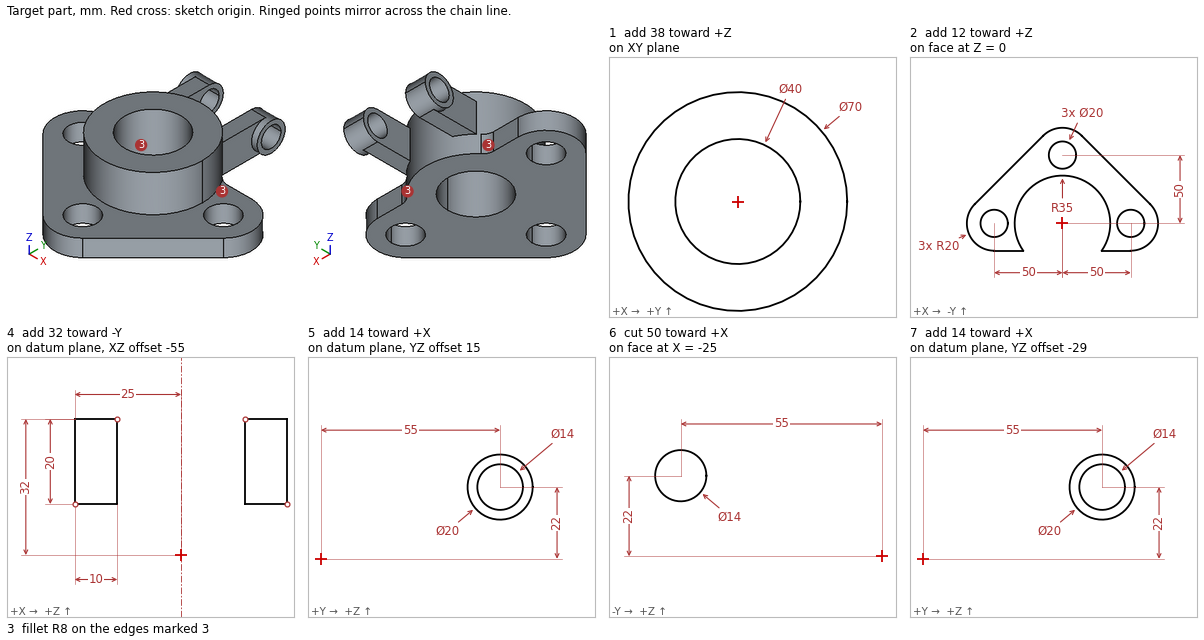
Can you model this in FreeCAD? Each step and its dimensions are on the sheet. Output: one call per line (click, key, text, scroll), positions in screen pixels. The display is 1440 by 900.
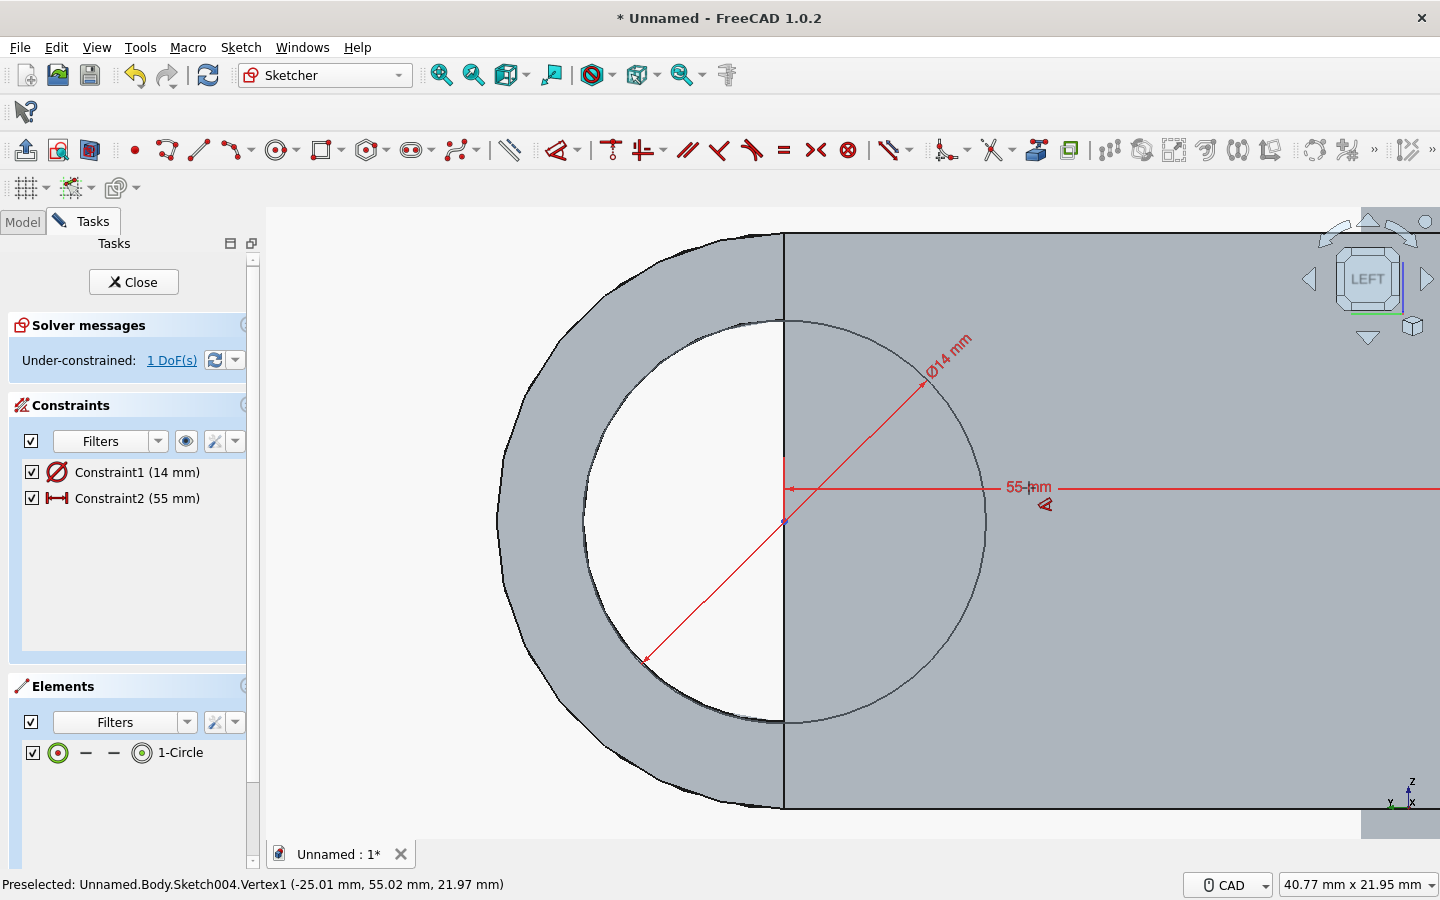
click(784, 522)
click(750, 667)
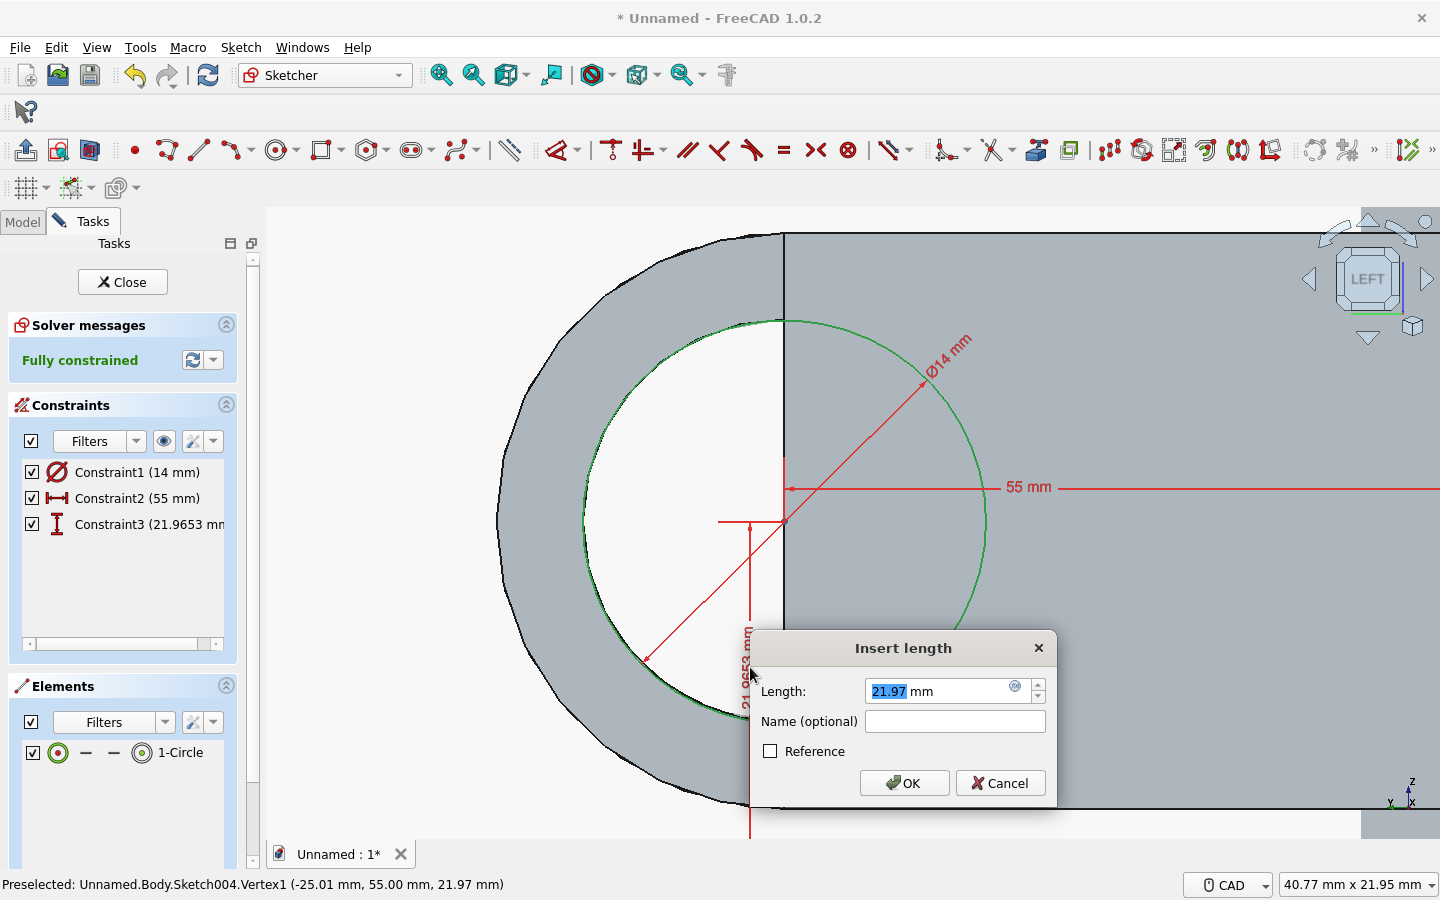
text(22)
key(Return)
key(Escape)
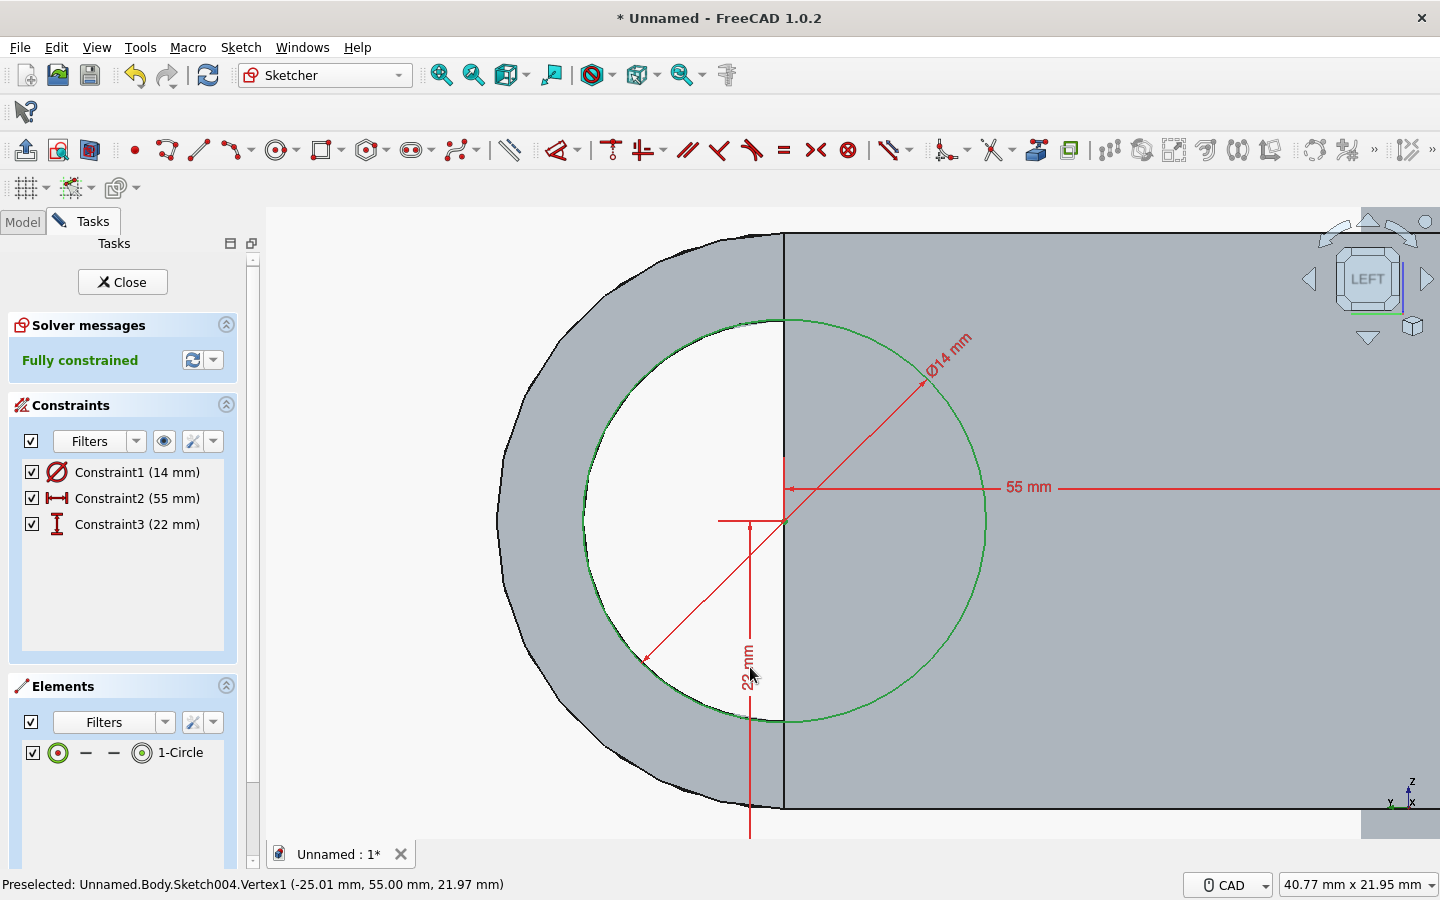
click(123, 282)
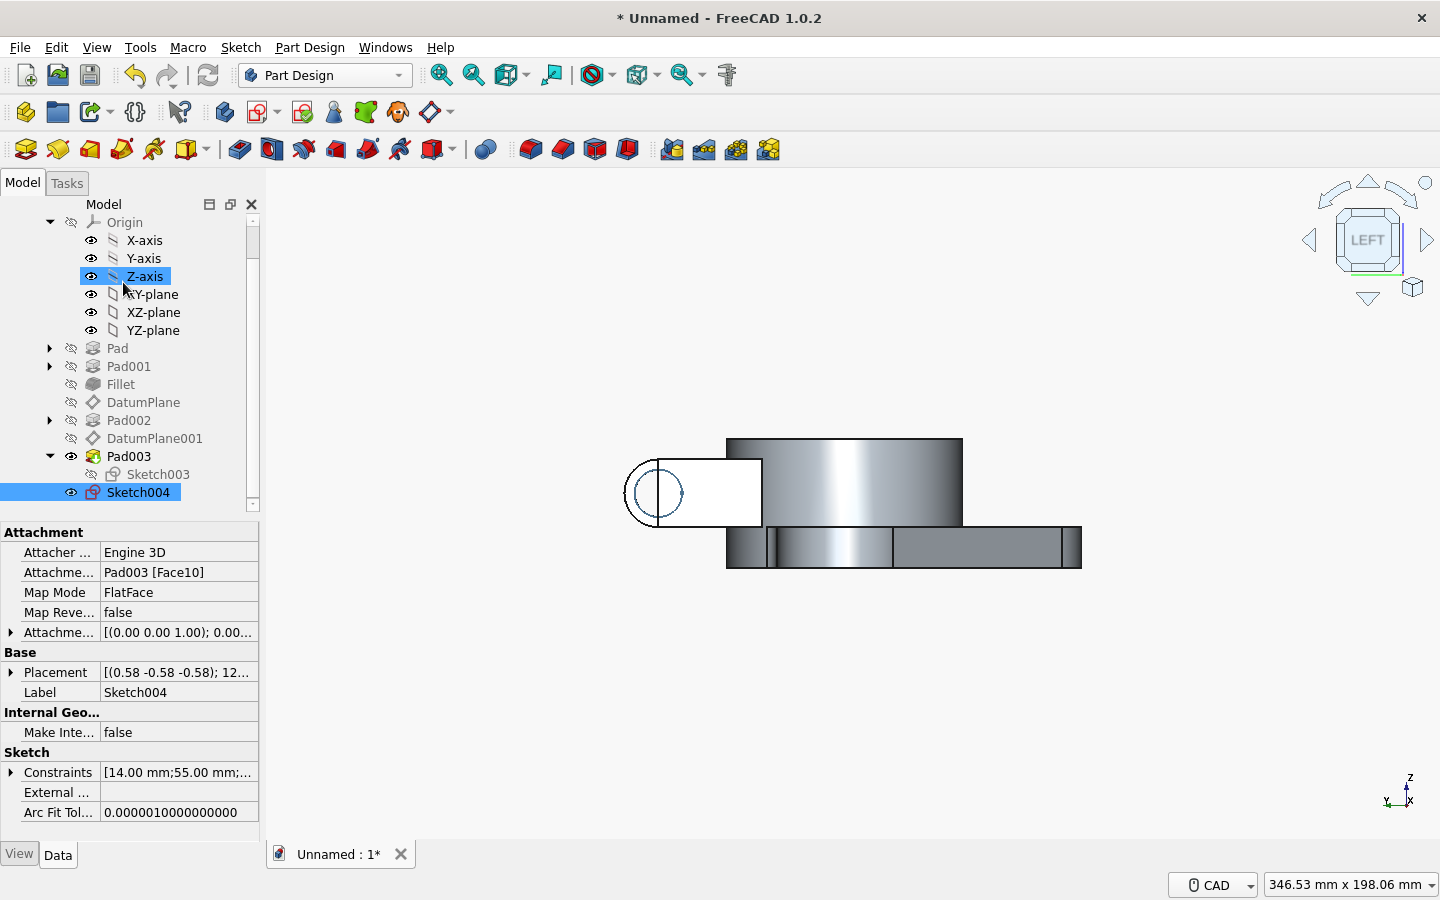
click(240, 150)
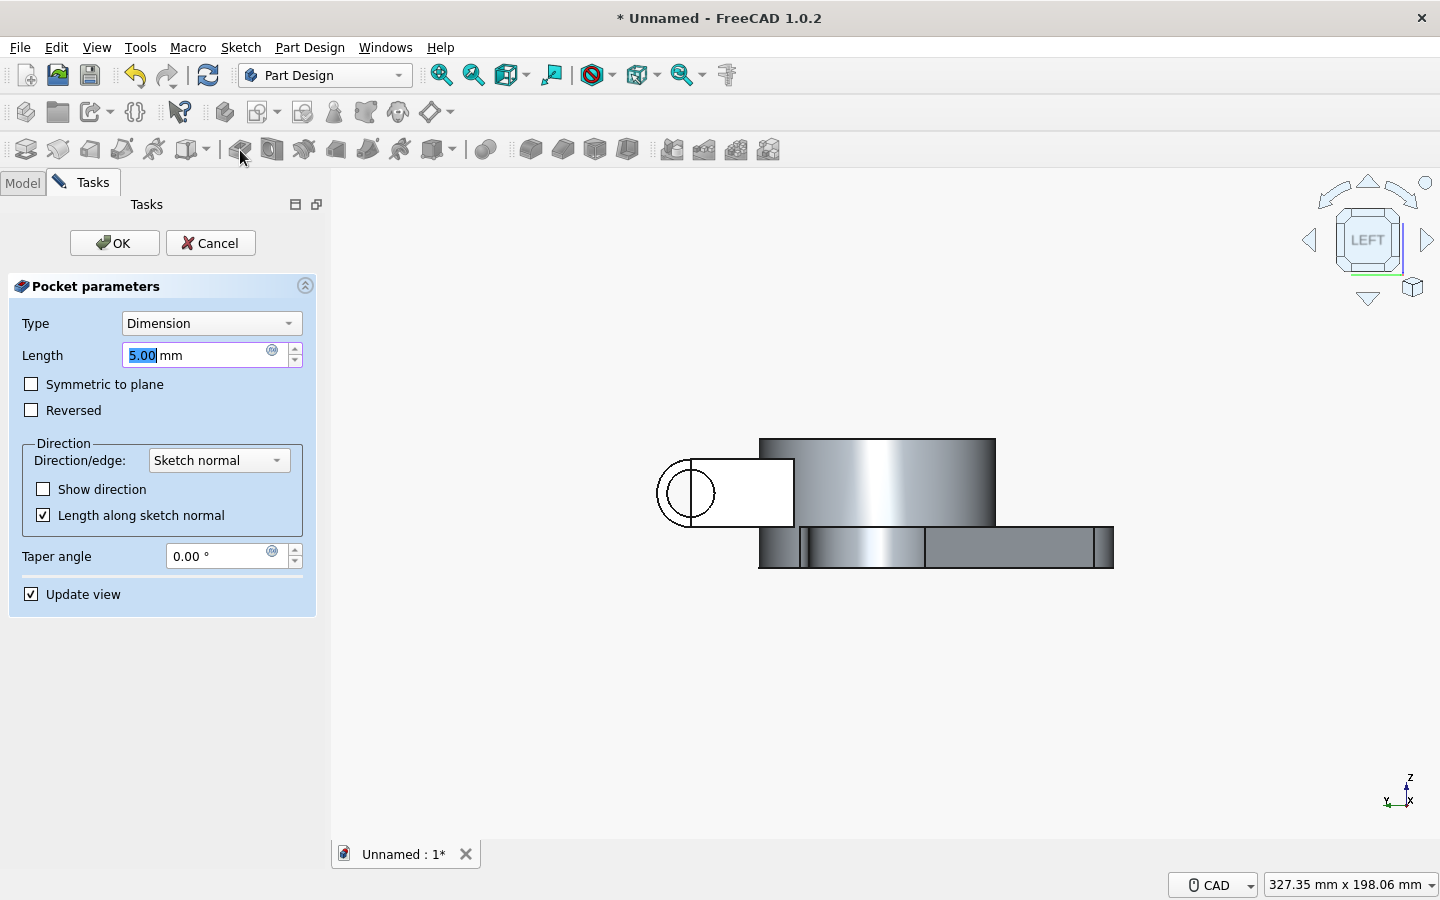
text(50)
key(Tab)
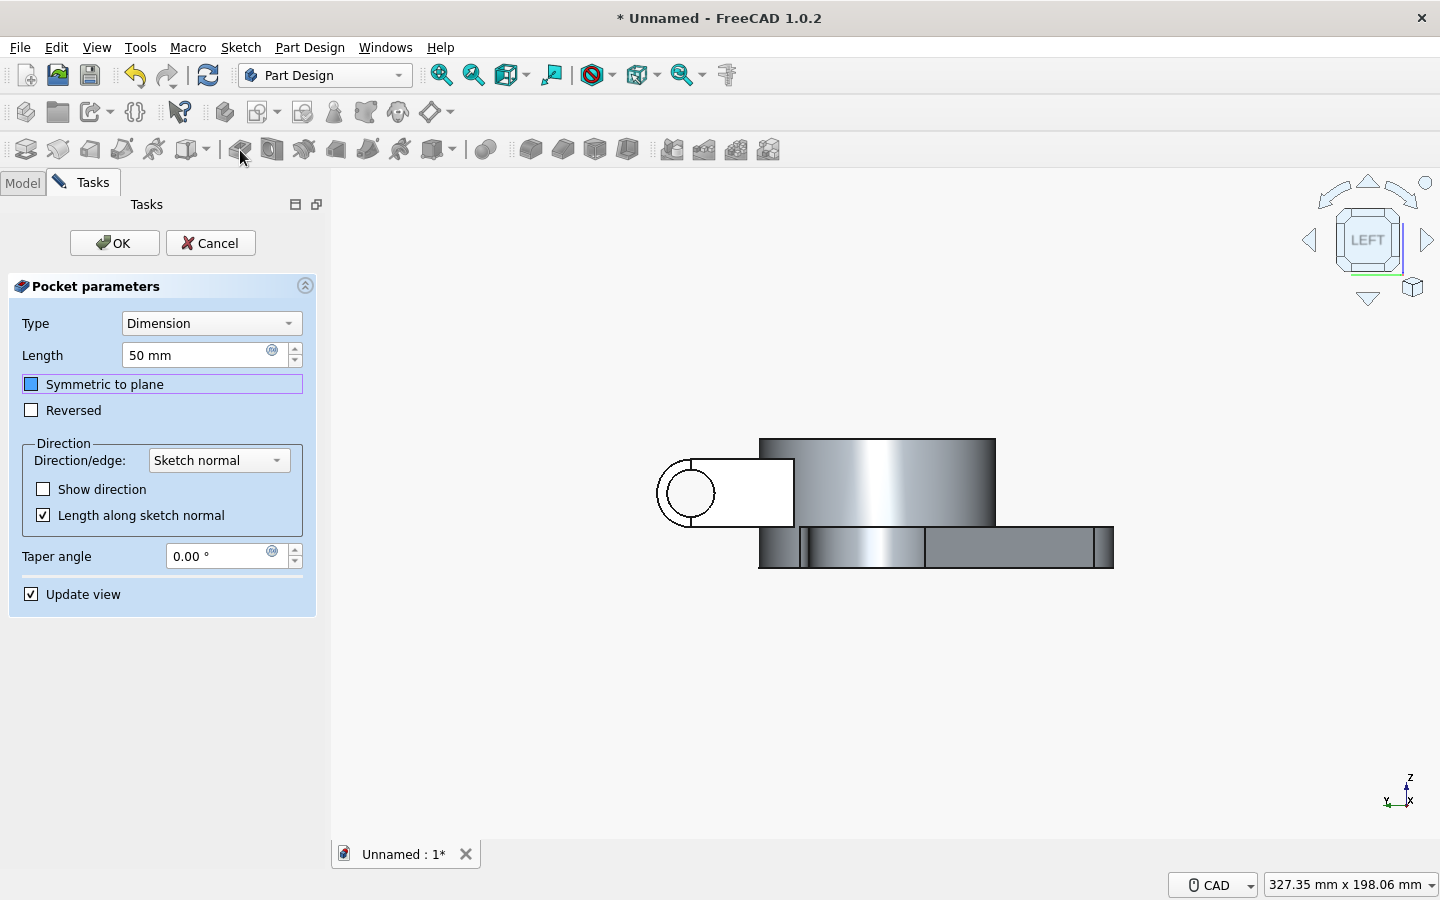
click(115, 243)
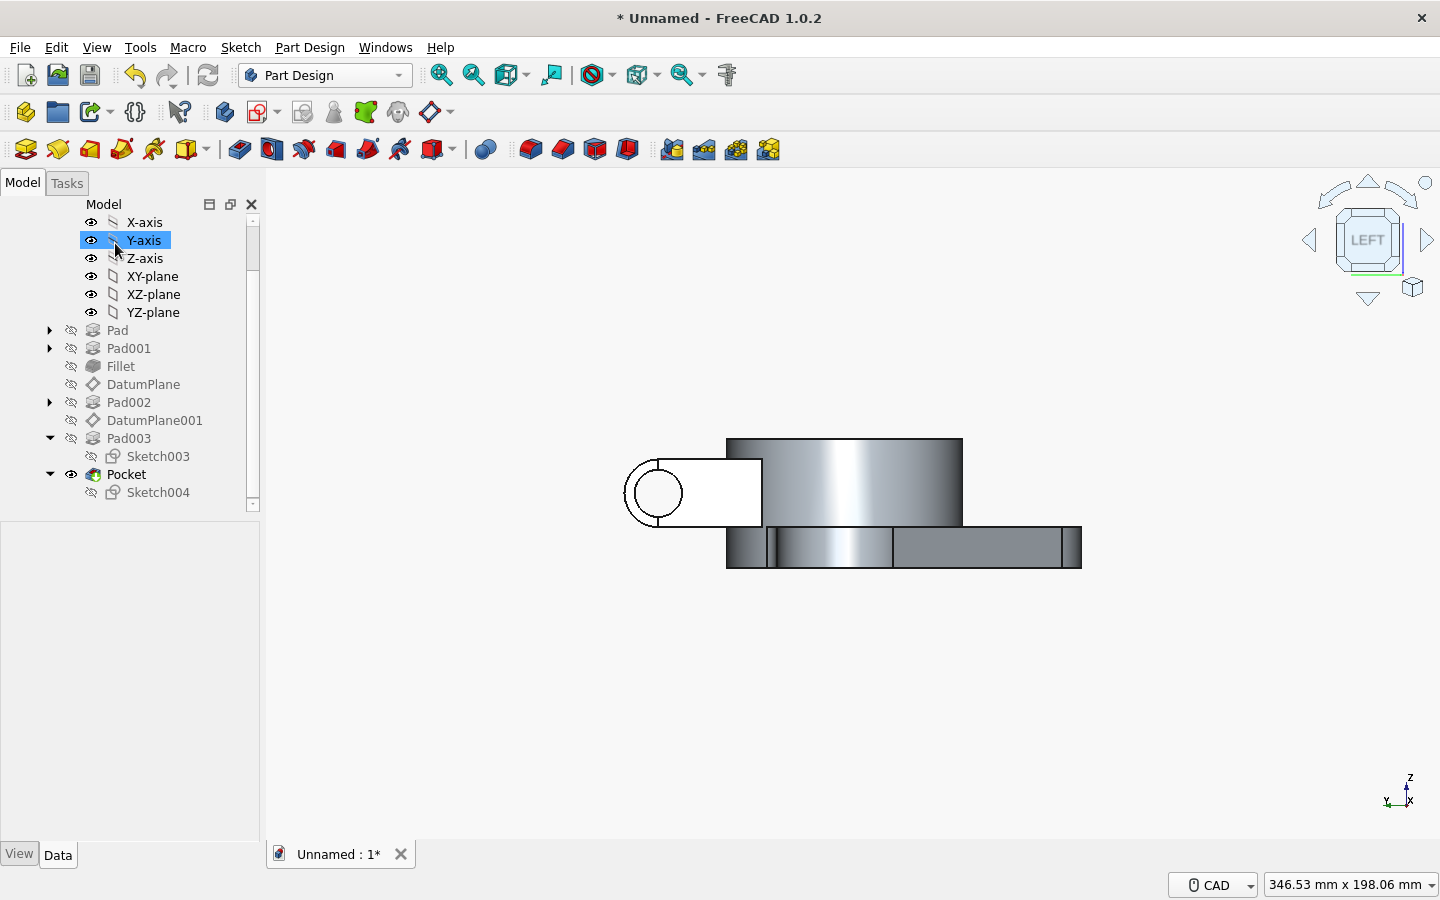
click(442, 76)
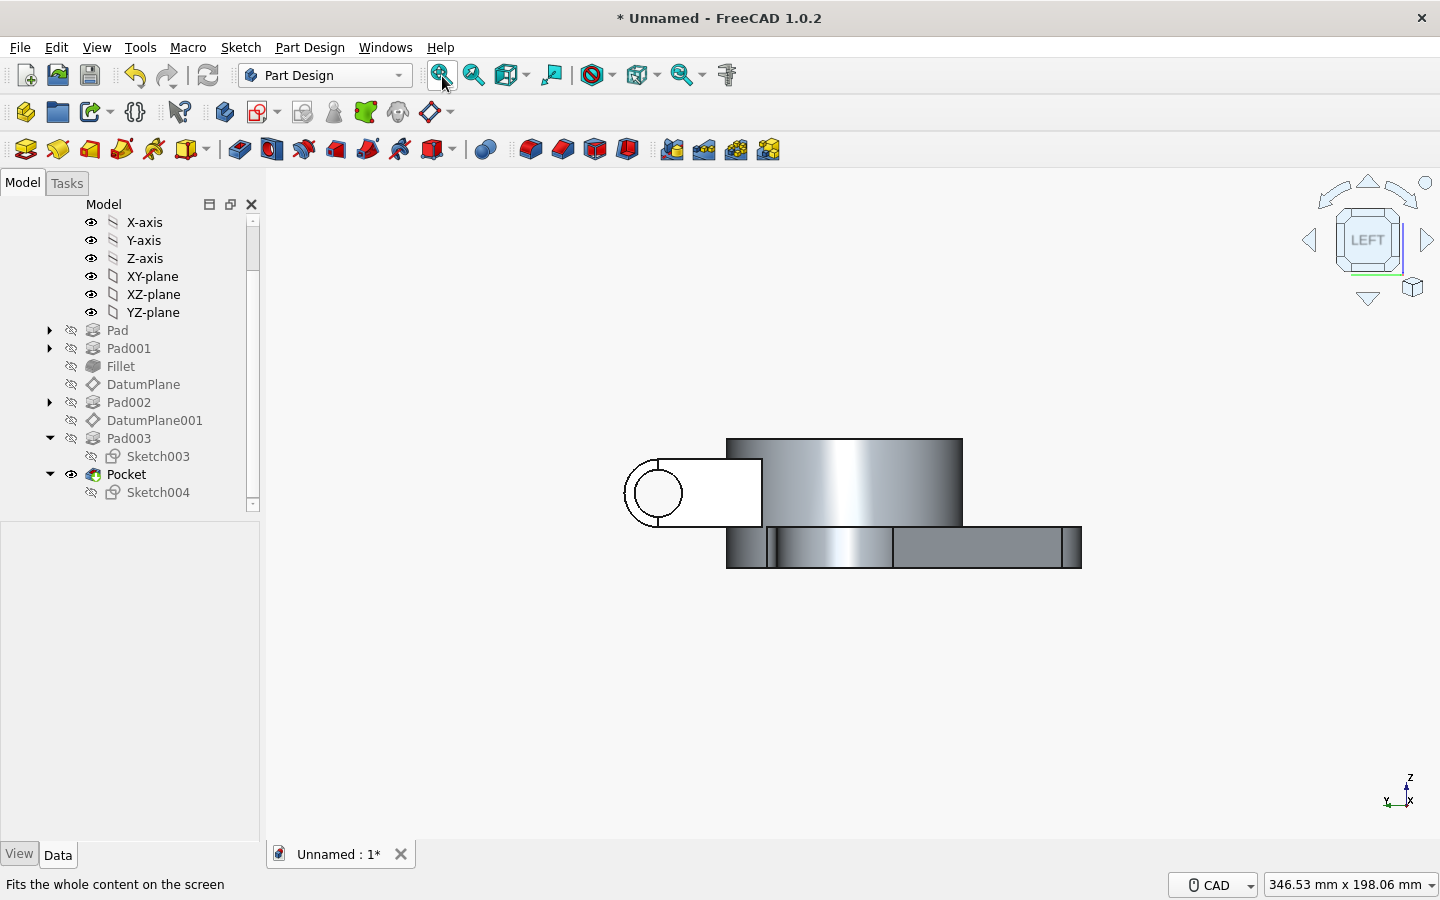
scroll(160, 362, down, 3)